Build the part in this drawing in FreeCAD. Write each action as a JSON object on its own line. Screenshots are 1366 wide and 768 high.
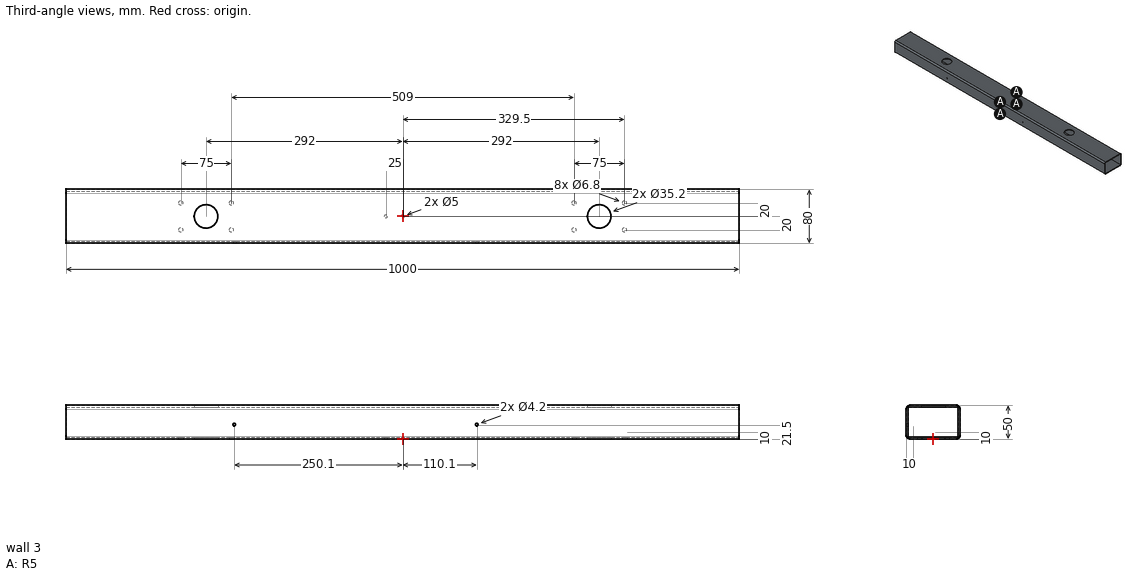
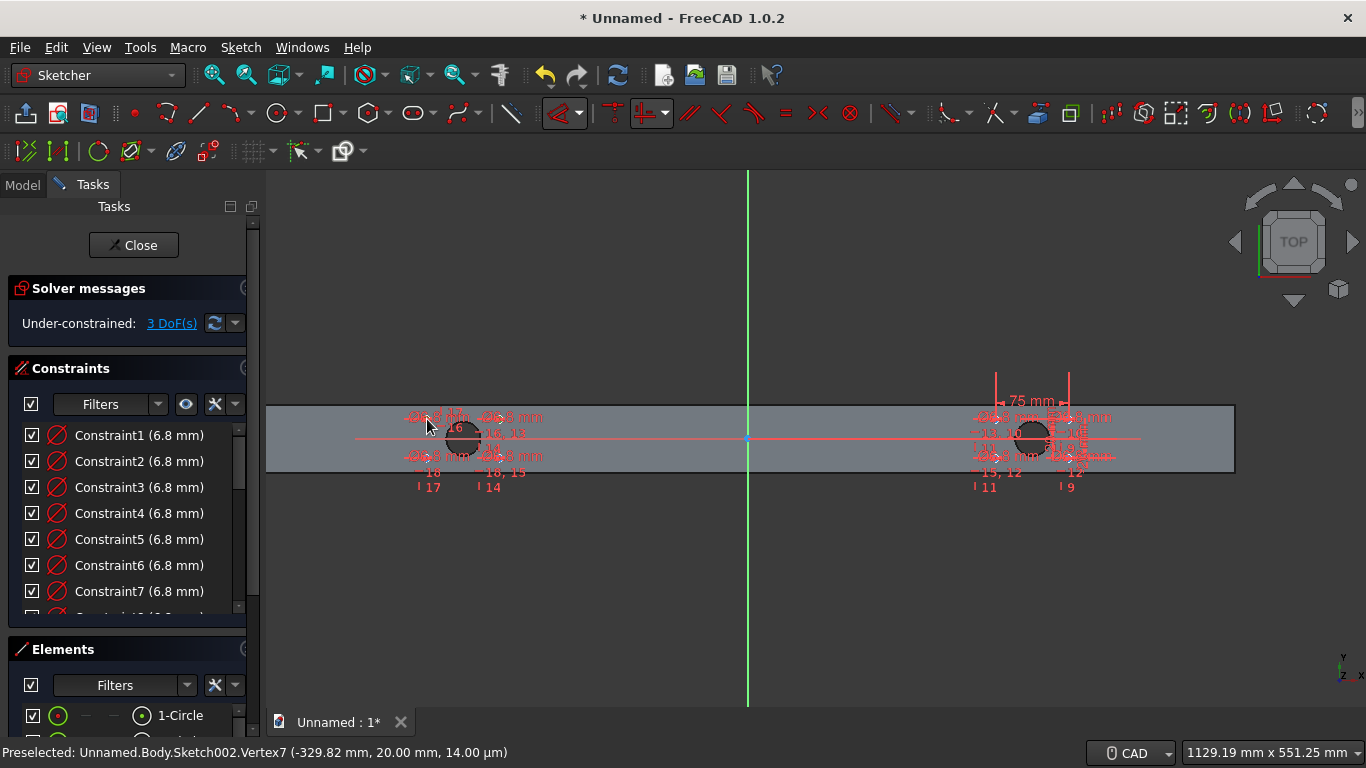
{"action": "key", "text": "l"}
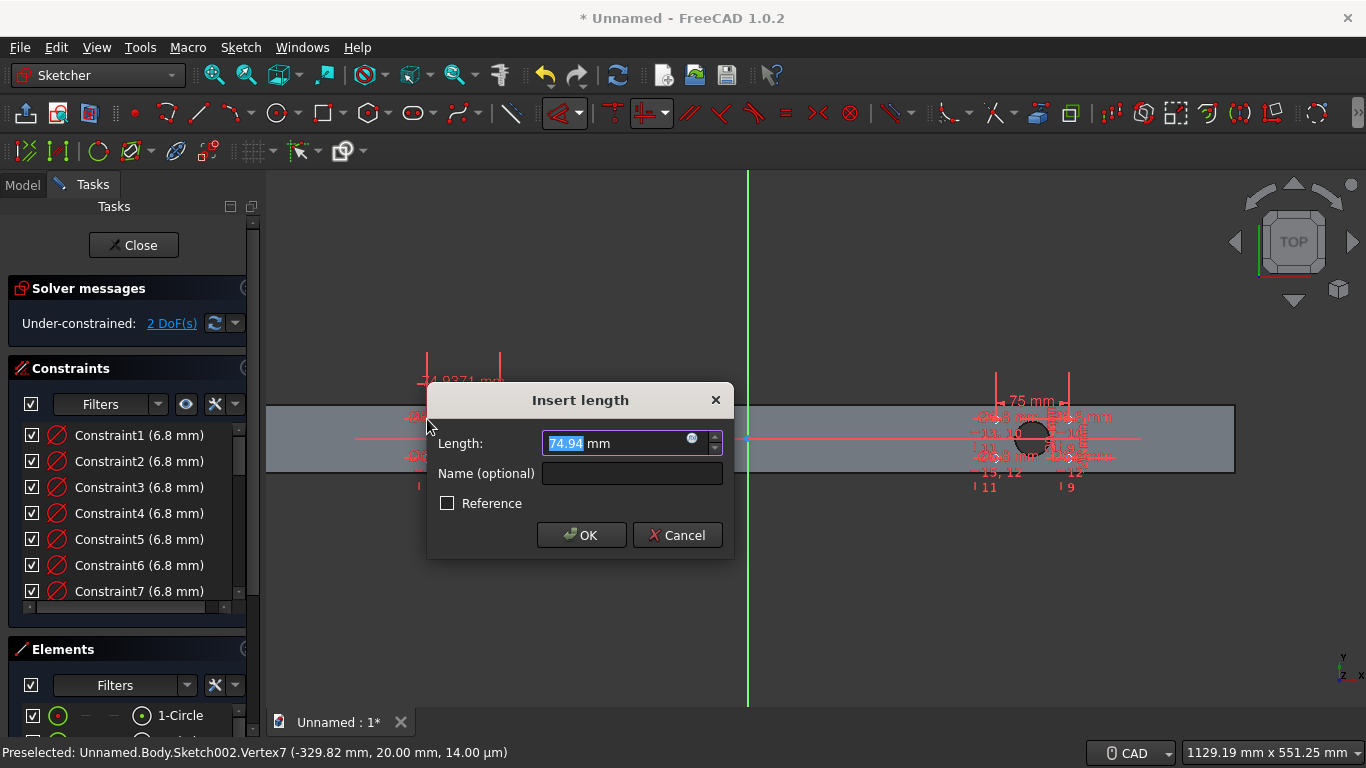
{"action": "type", "text": "75"}
{"action": "key", "text": "Return"}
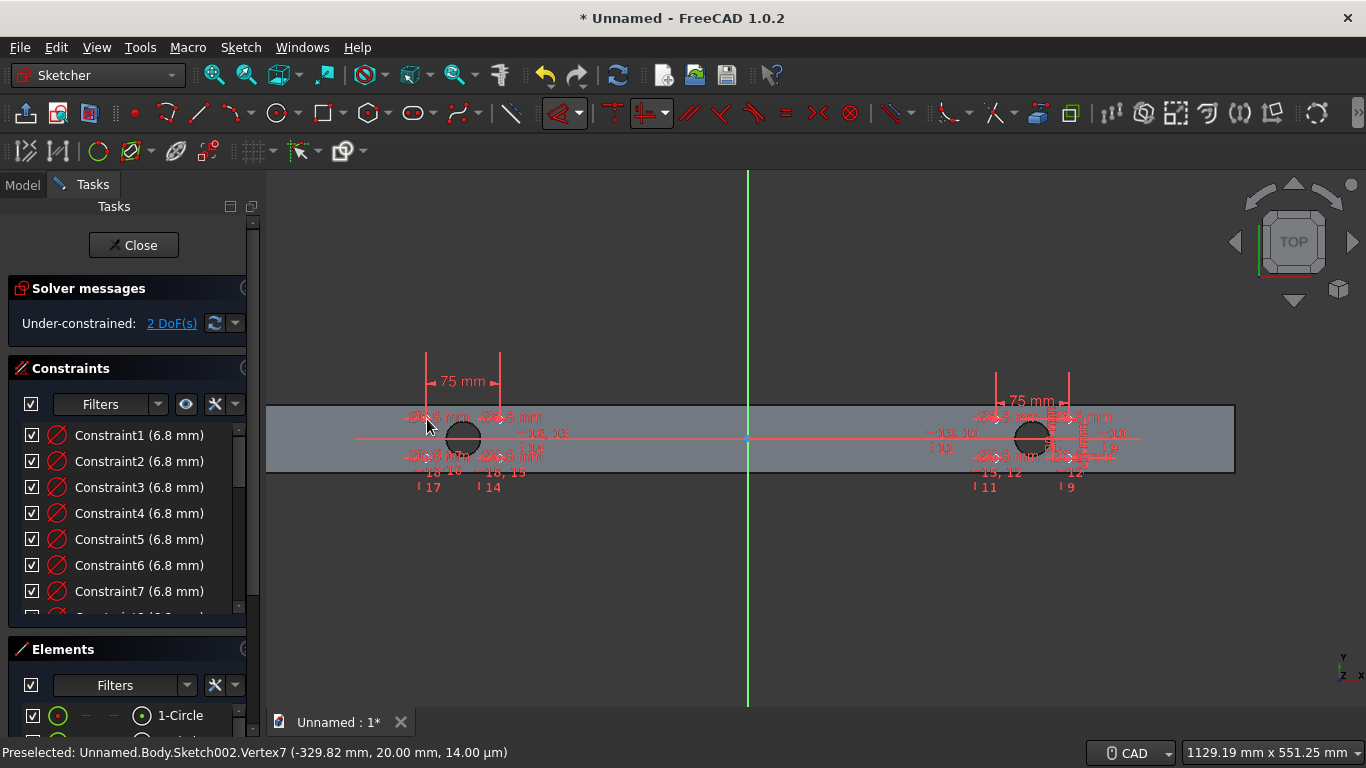
{"action": "left_click", "coordinate": [996, 419]}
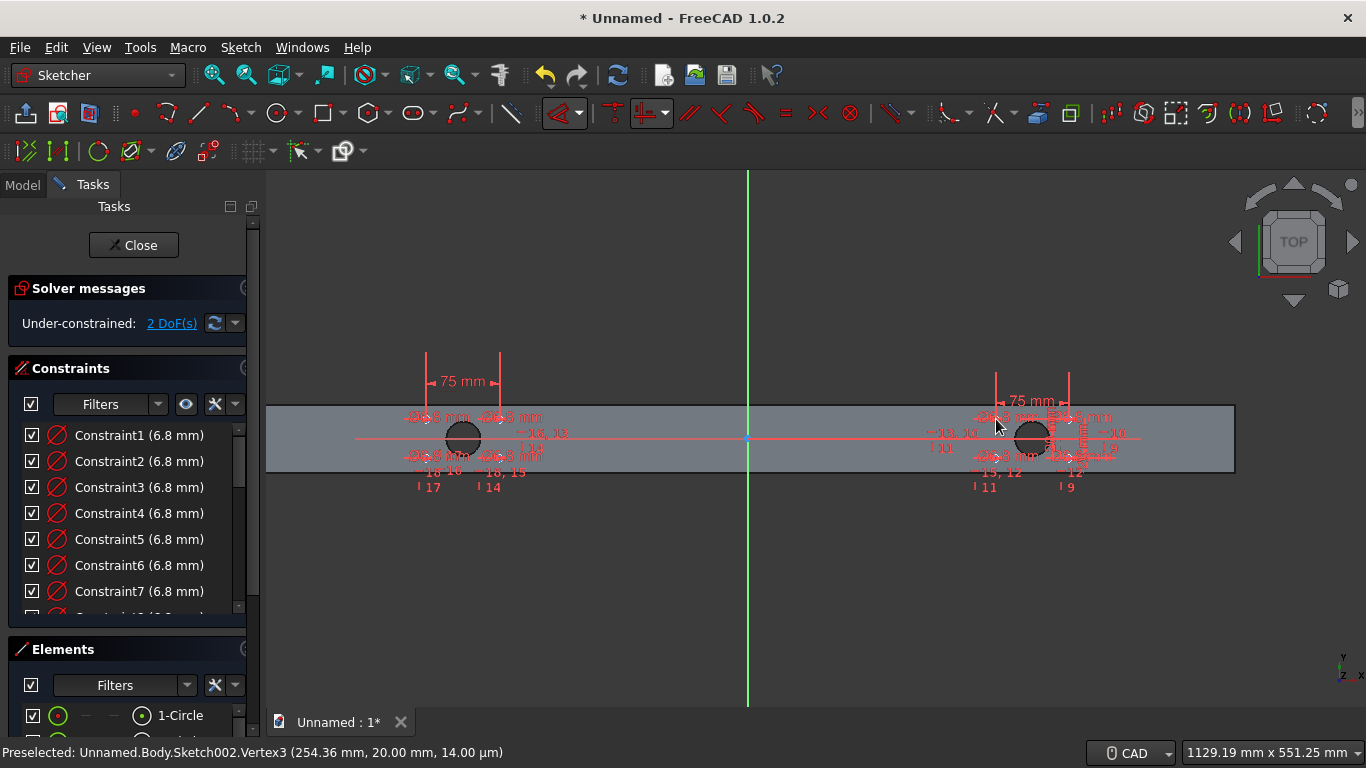
{"action": "left_click", "coordinate": [500, 419]}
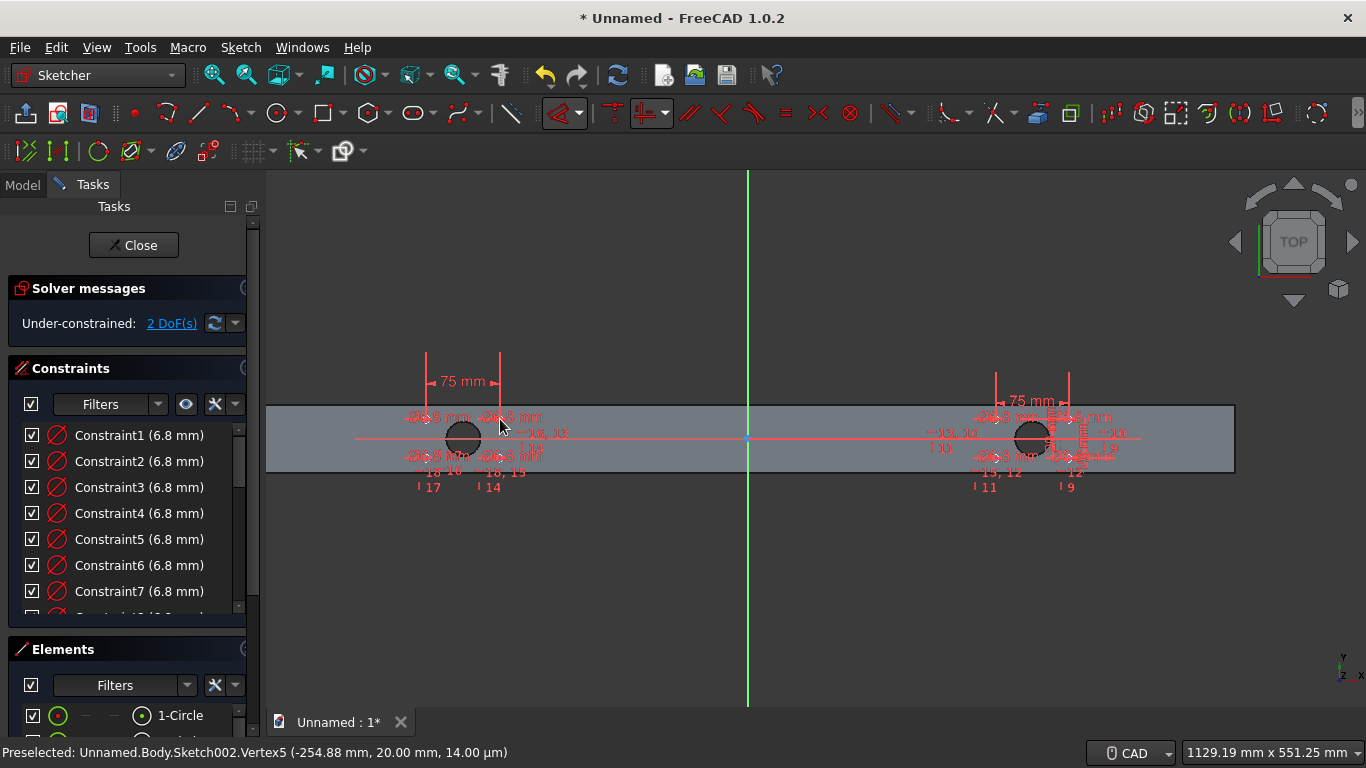
{"action": "key", "text": "l"}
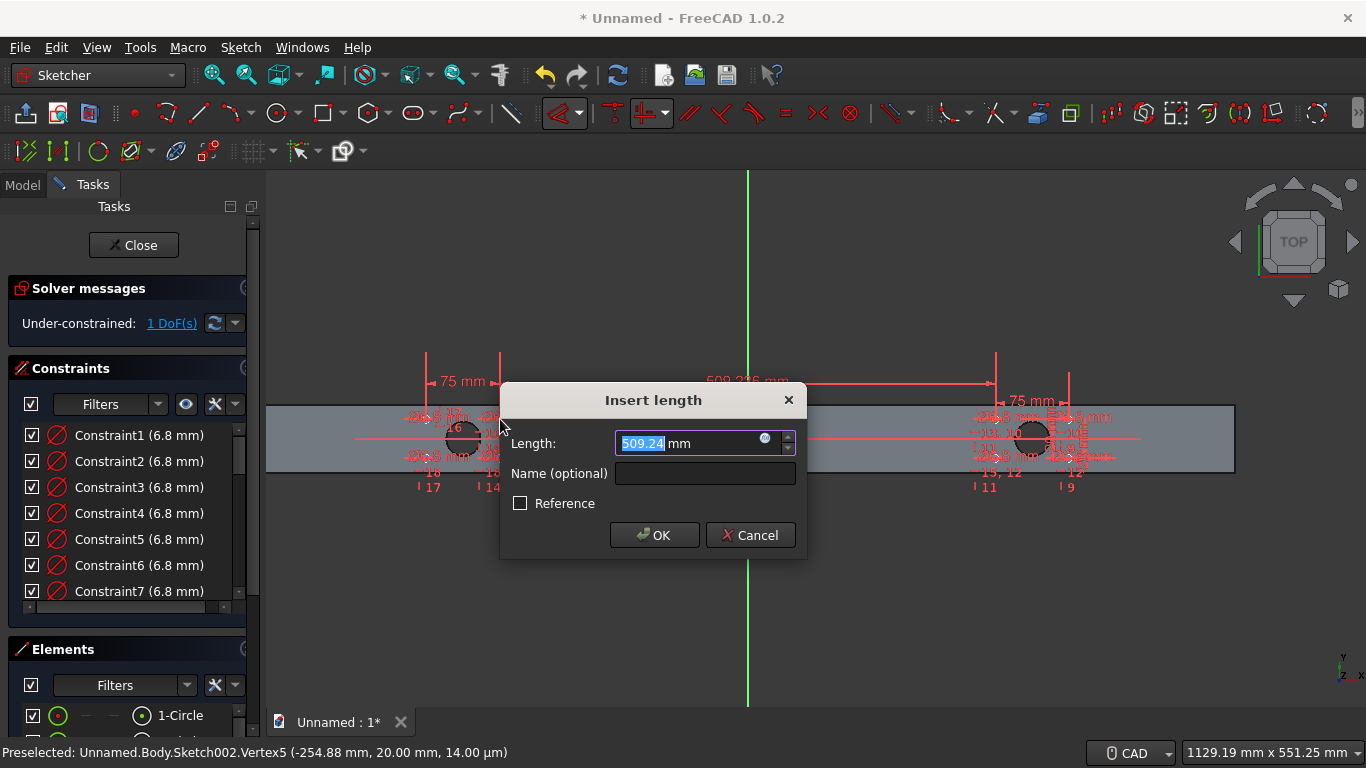
{"action": "type", "text": "509"}
{"action": "key", "text": "Return"}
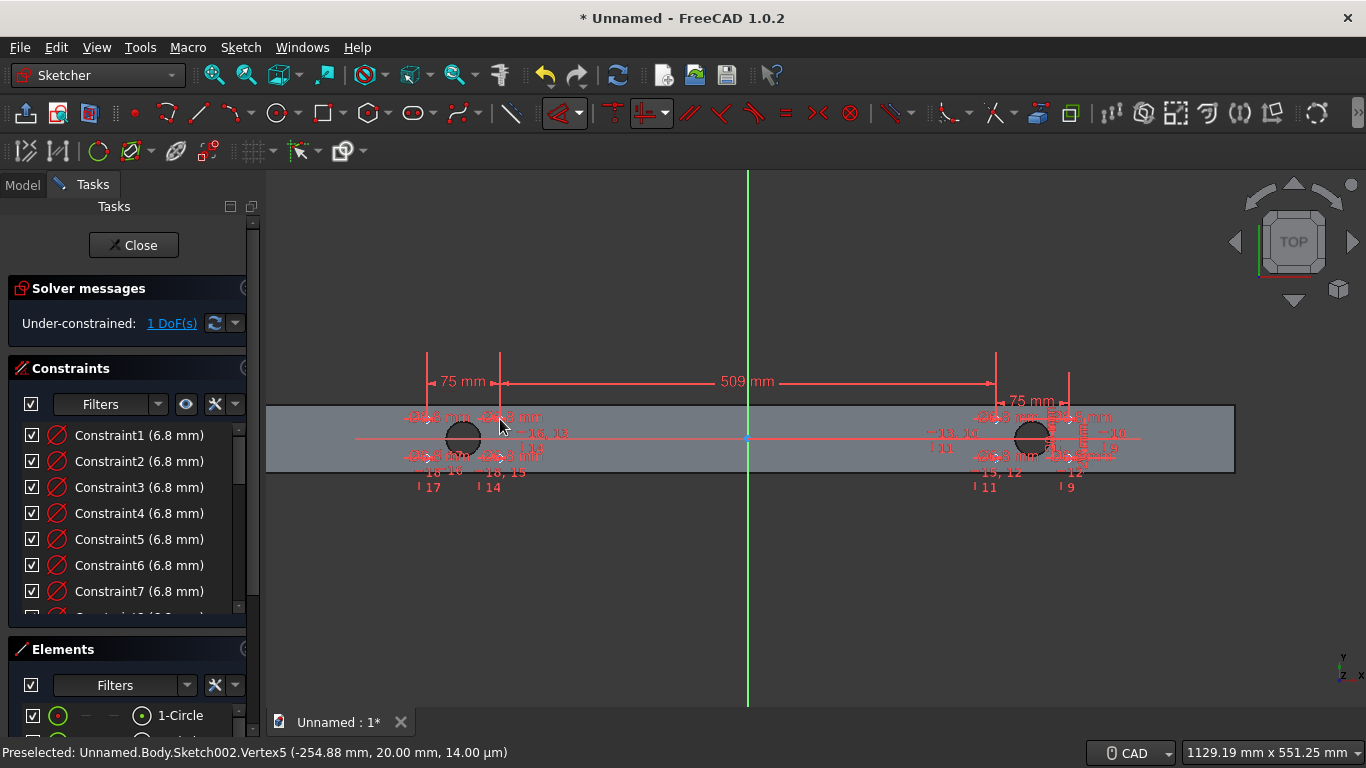
{"action": "left_click", "coordinate": [1069, 419]}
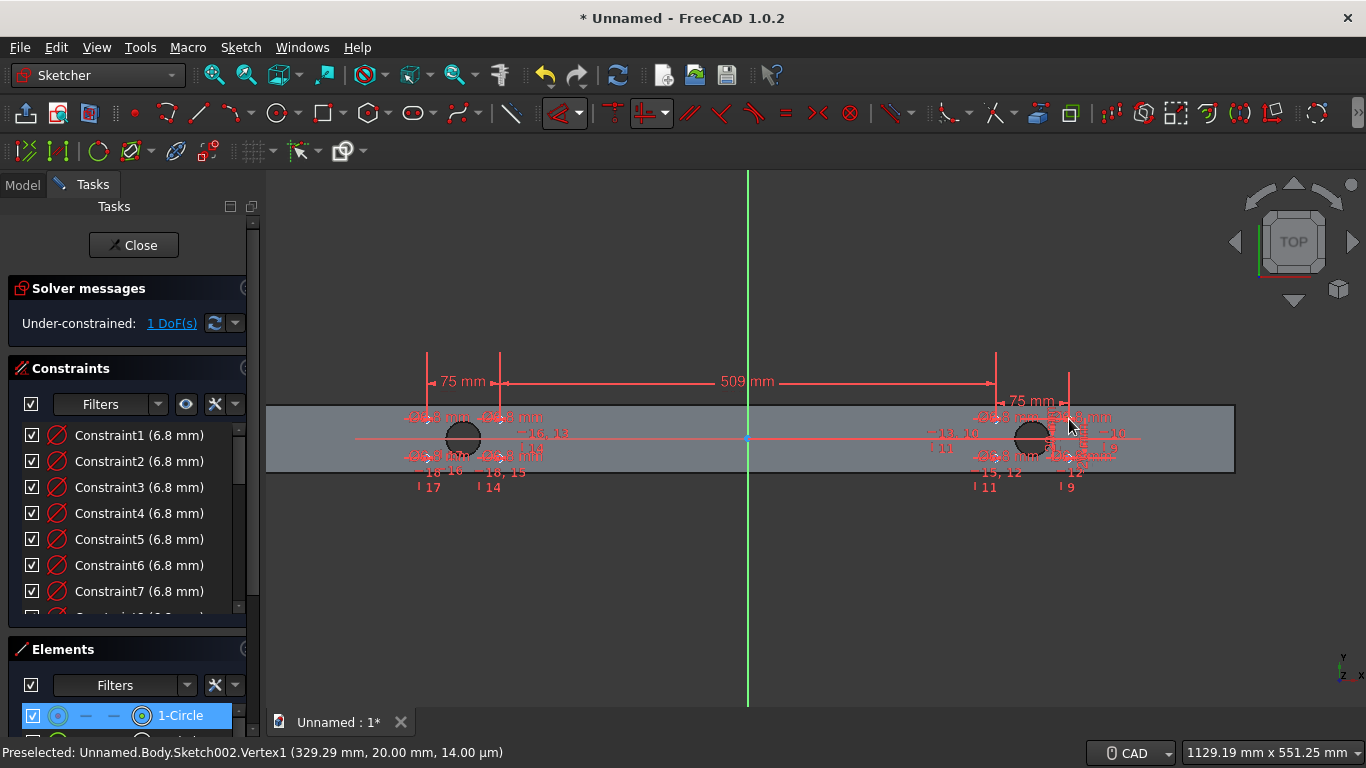
{"action": "key", "text": "l"}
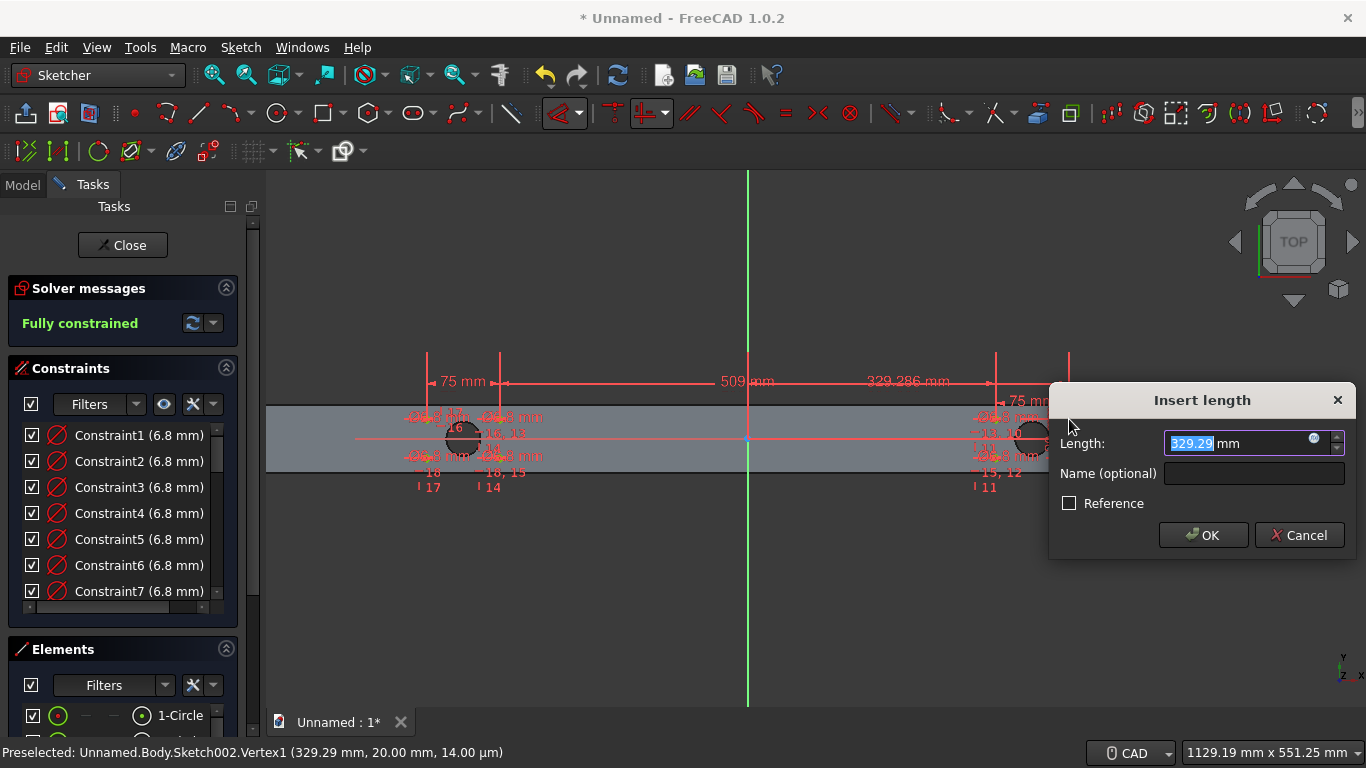
{"action": "type", "text": "329.5"}
{"action": "key", "text": "Return"}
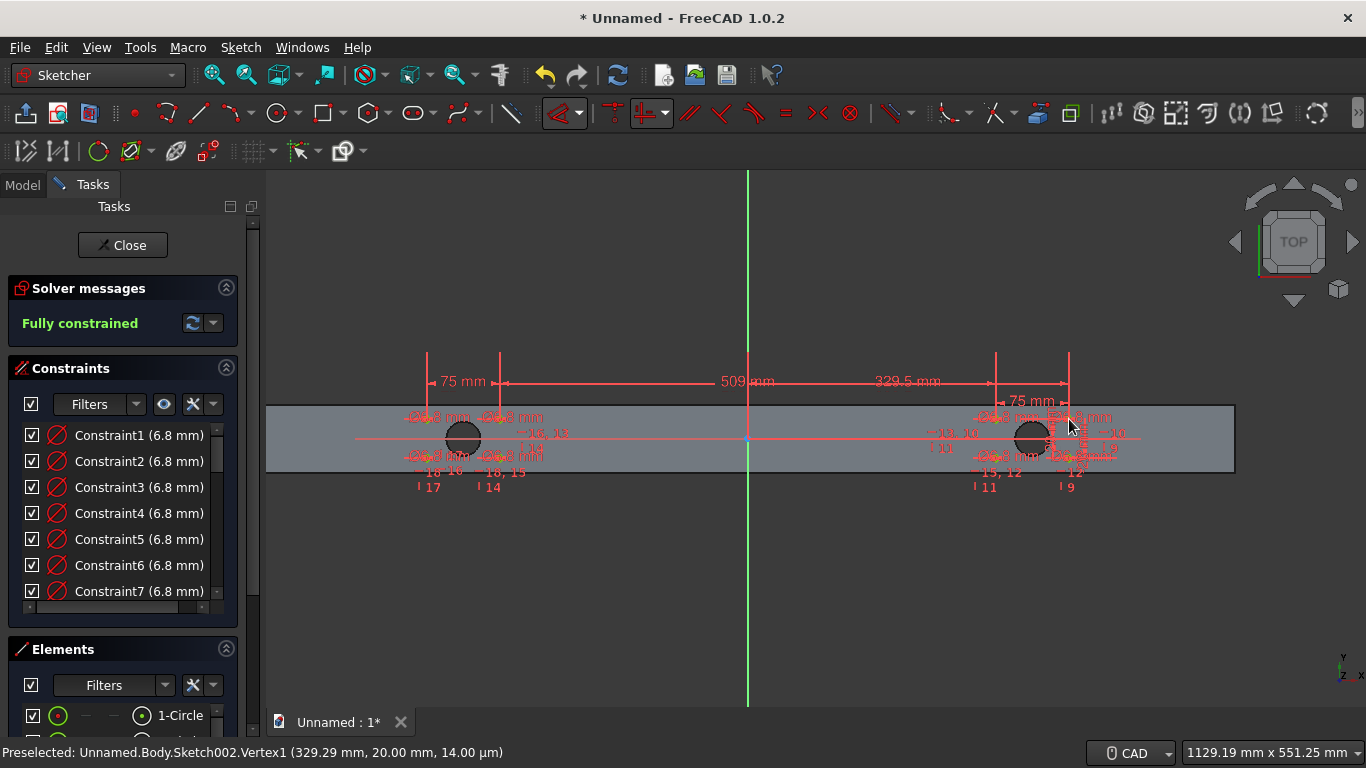
{"action": "left_click", "coordinate": [123, 245]}